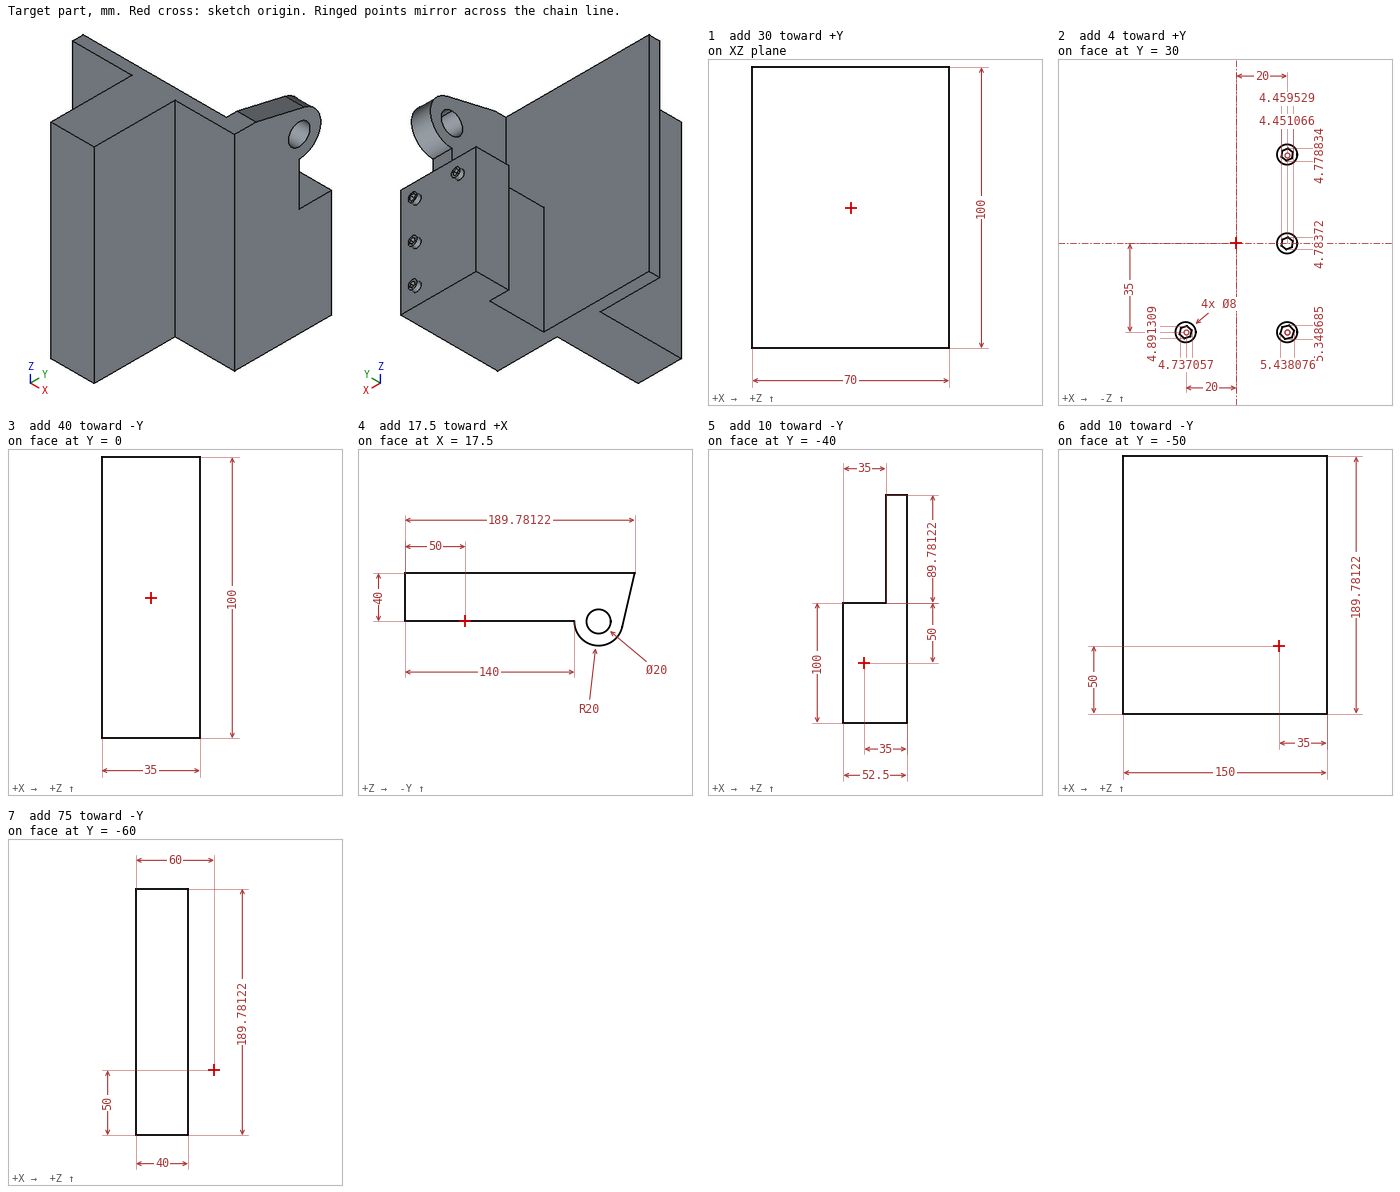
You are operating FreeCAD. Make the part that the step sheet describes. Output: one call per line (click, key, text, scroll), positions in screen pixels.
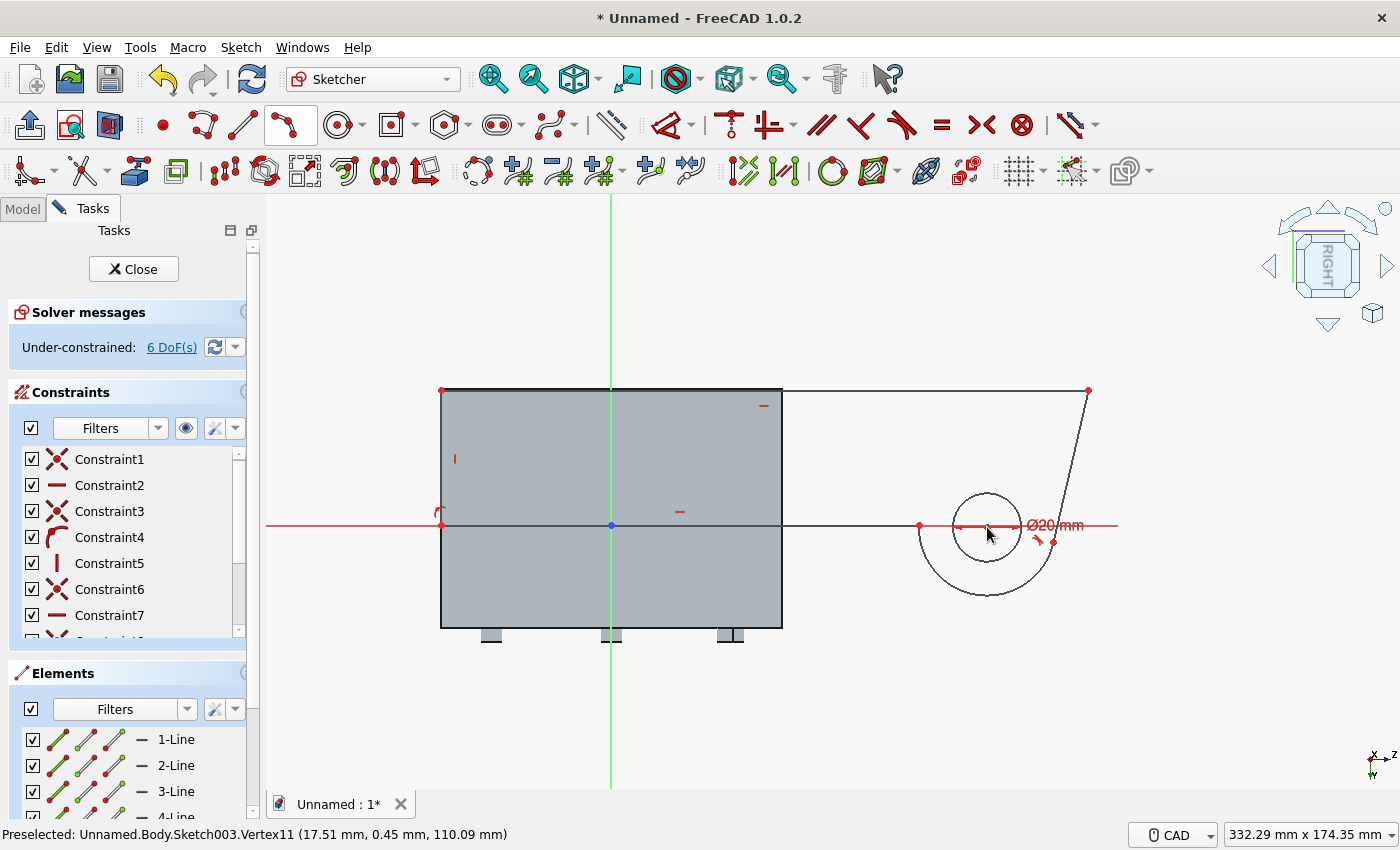
click(361, 526)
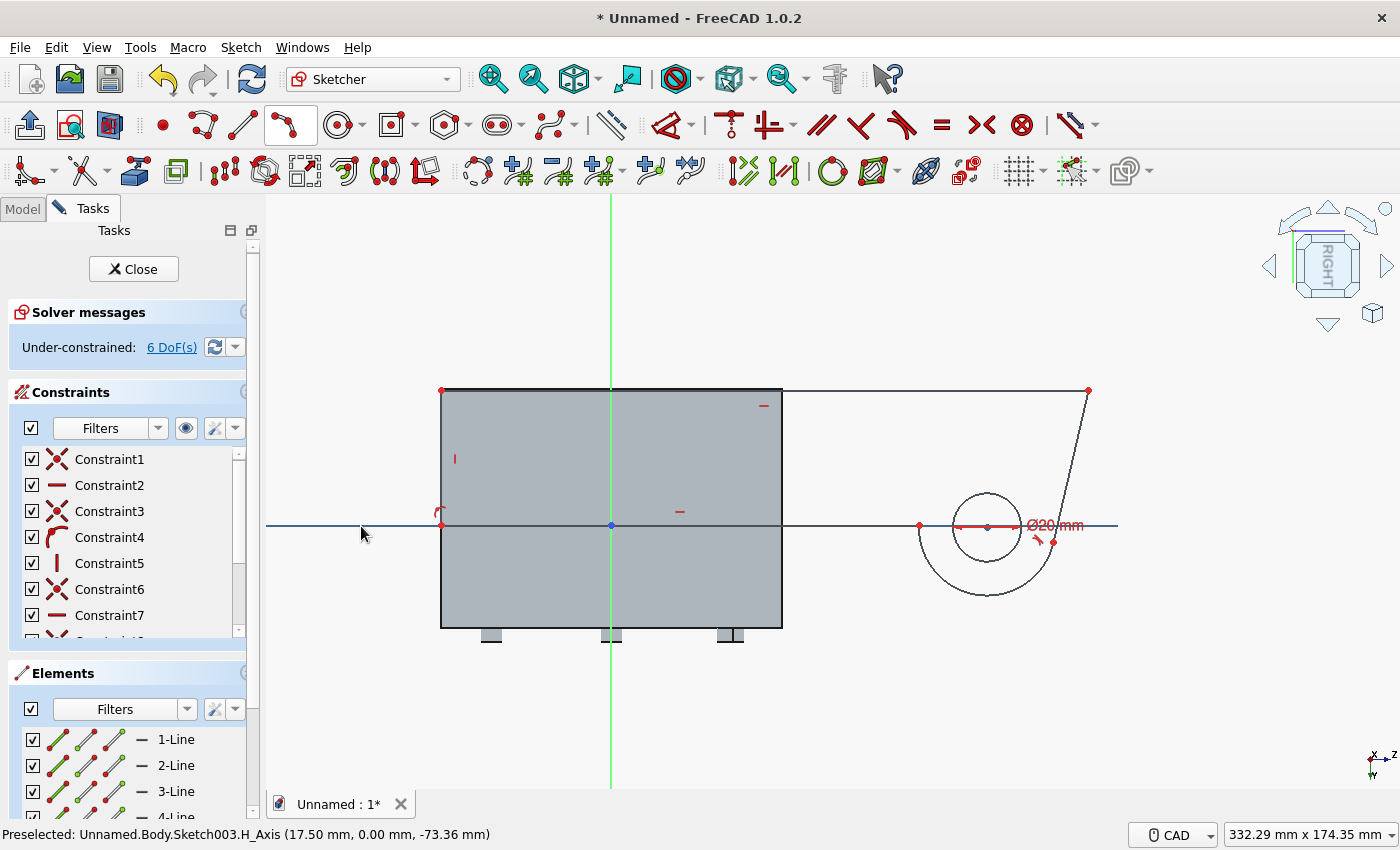
click(730, 126)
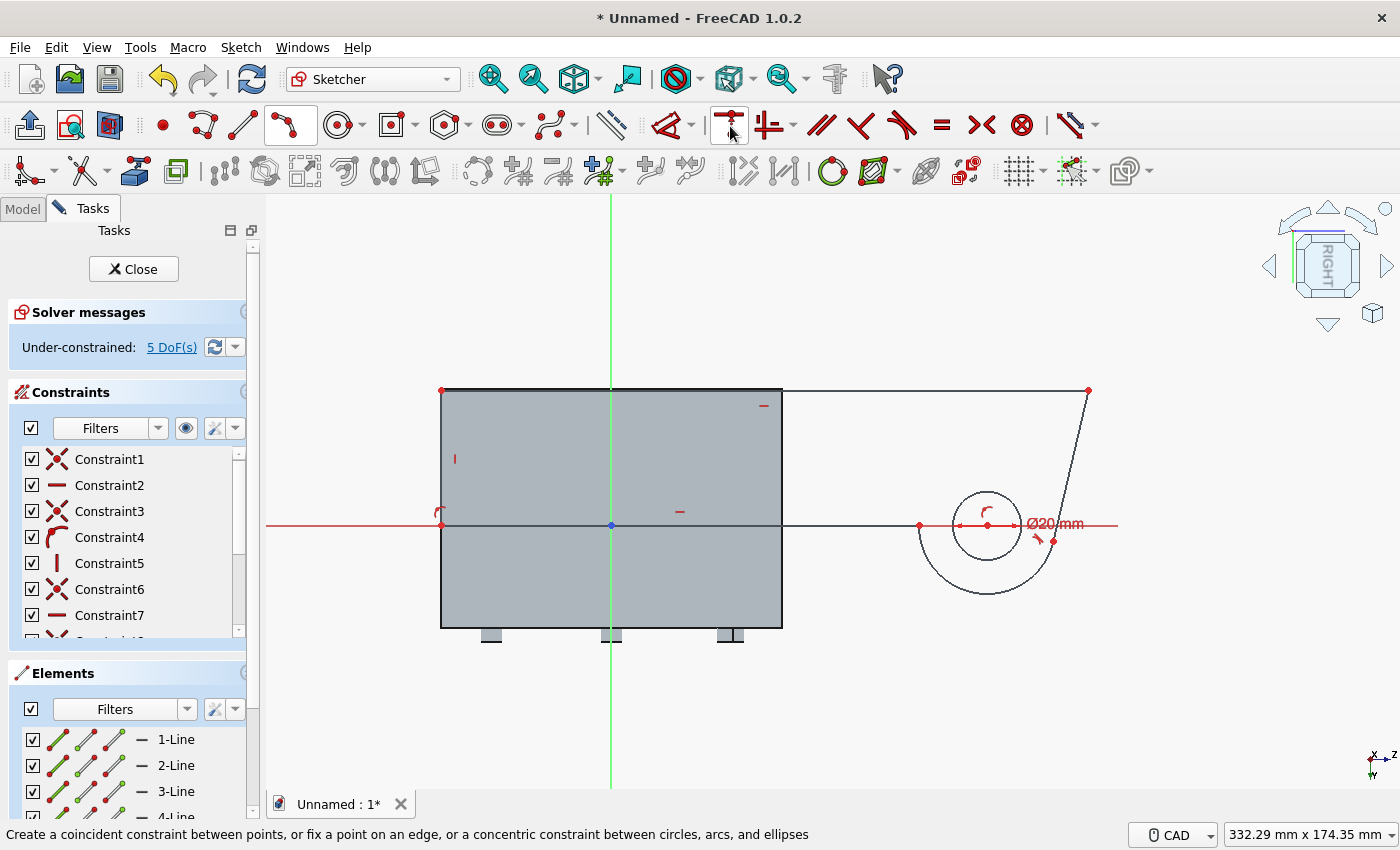
key(d)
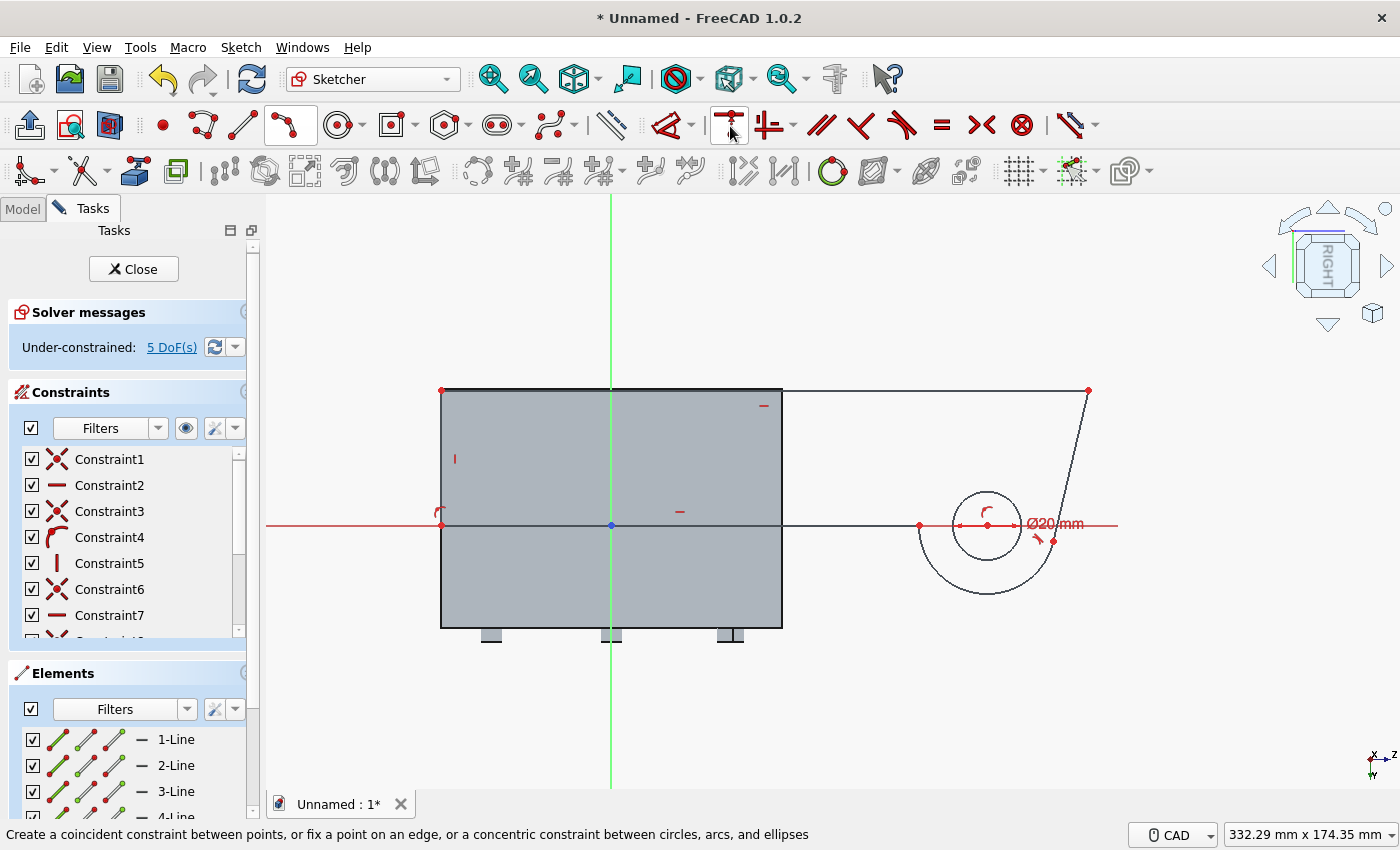
click(943, 578)
click(922, 602)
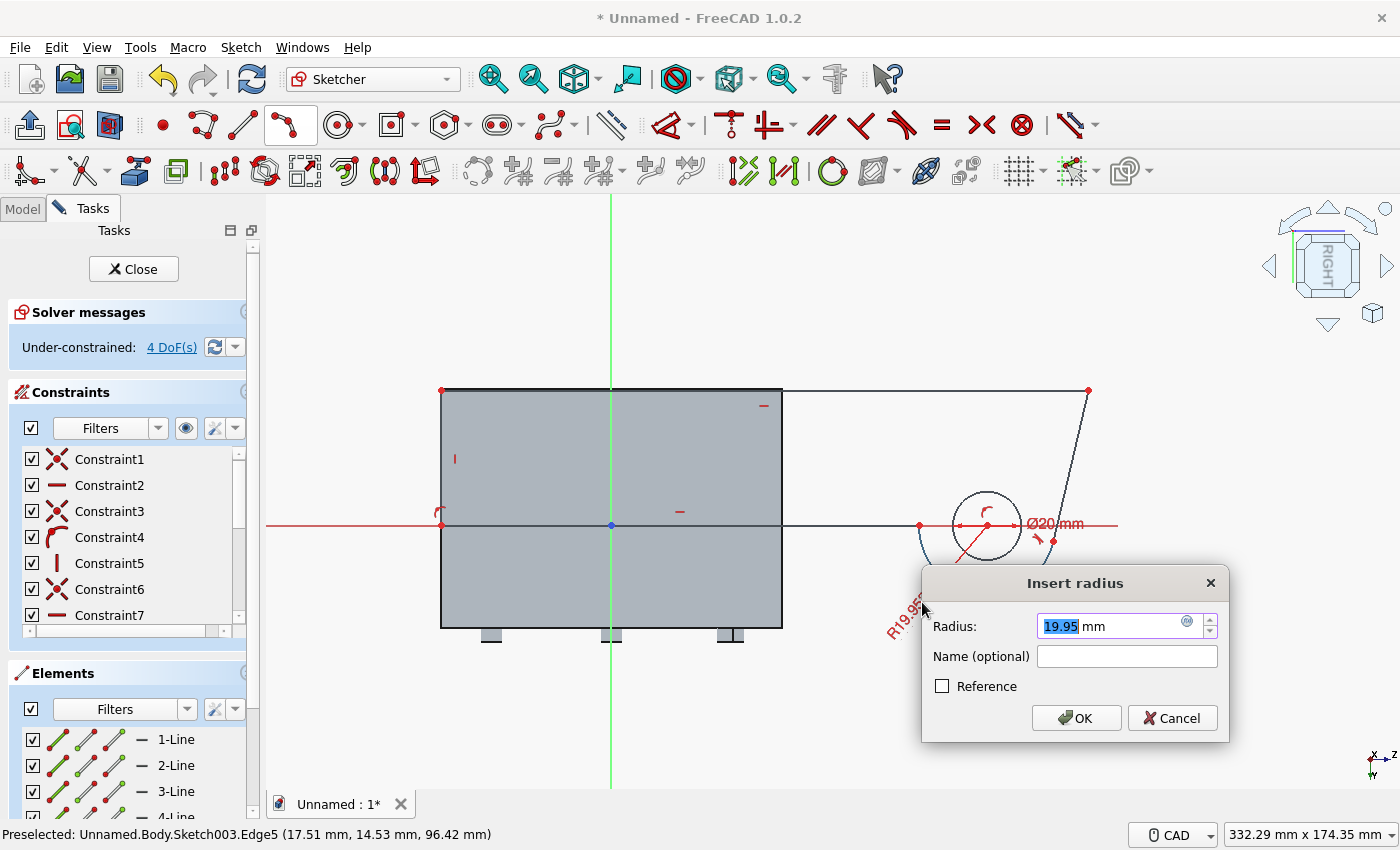
text(20)
key(Return)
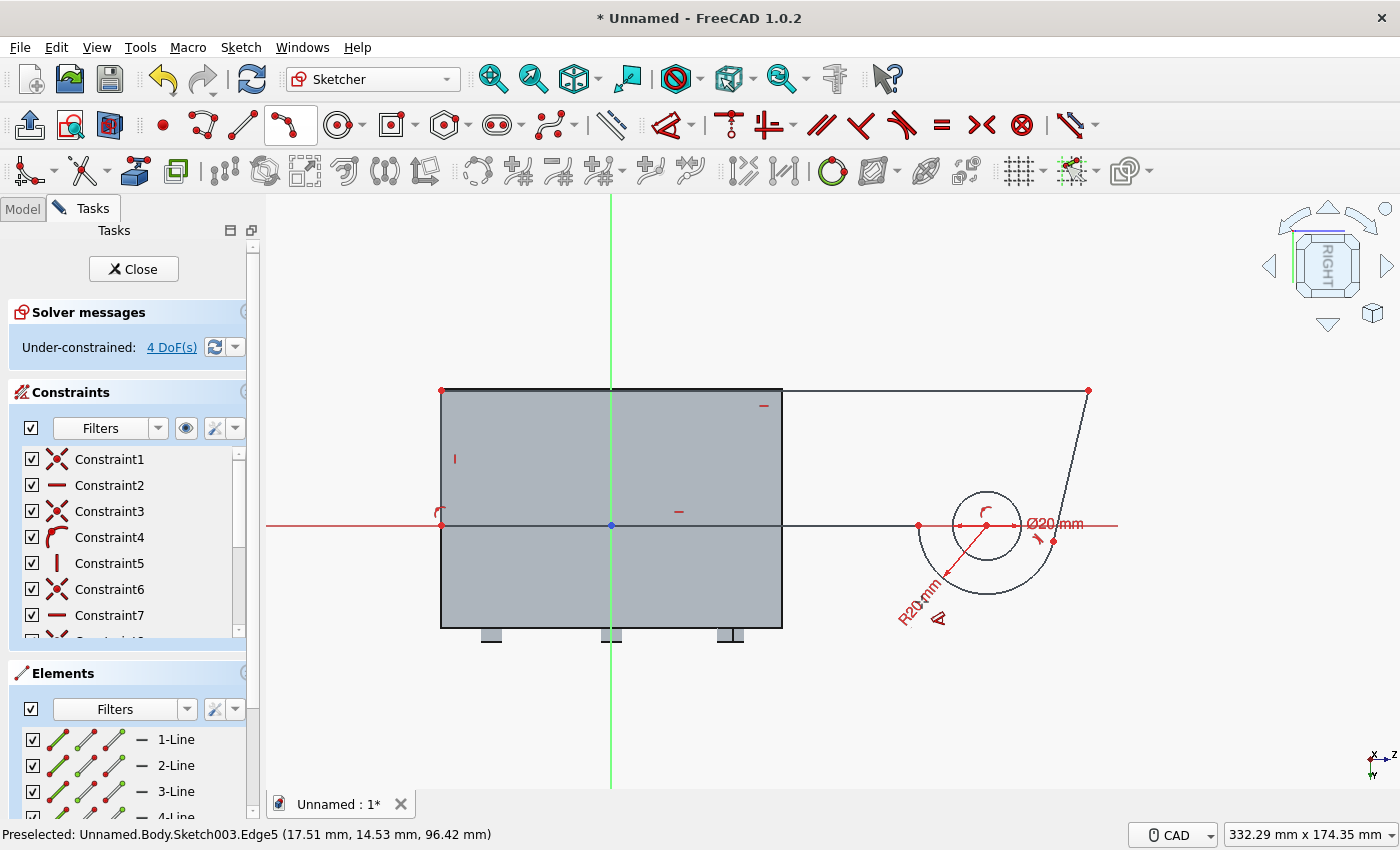
click(441, 431)
click(407, 458)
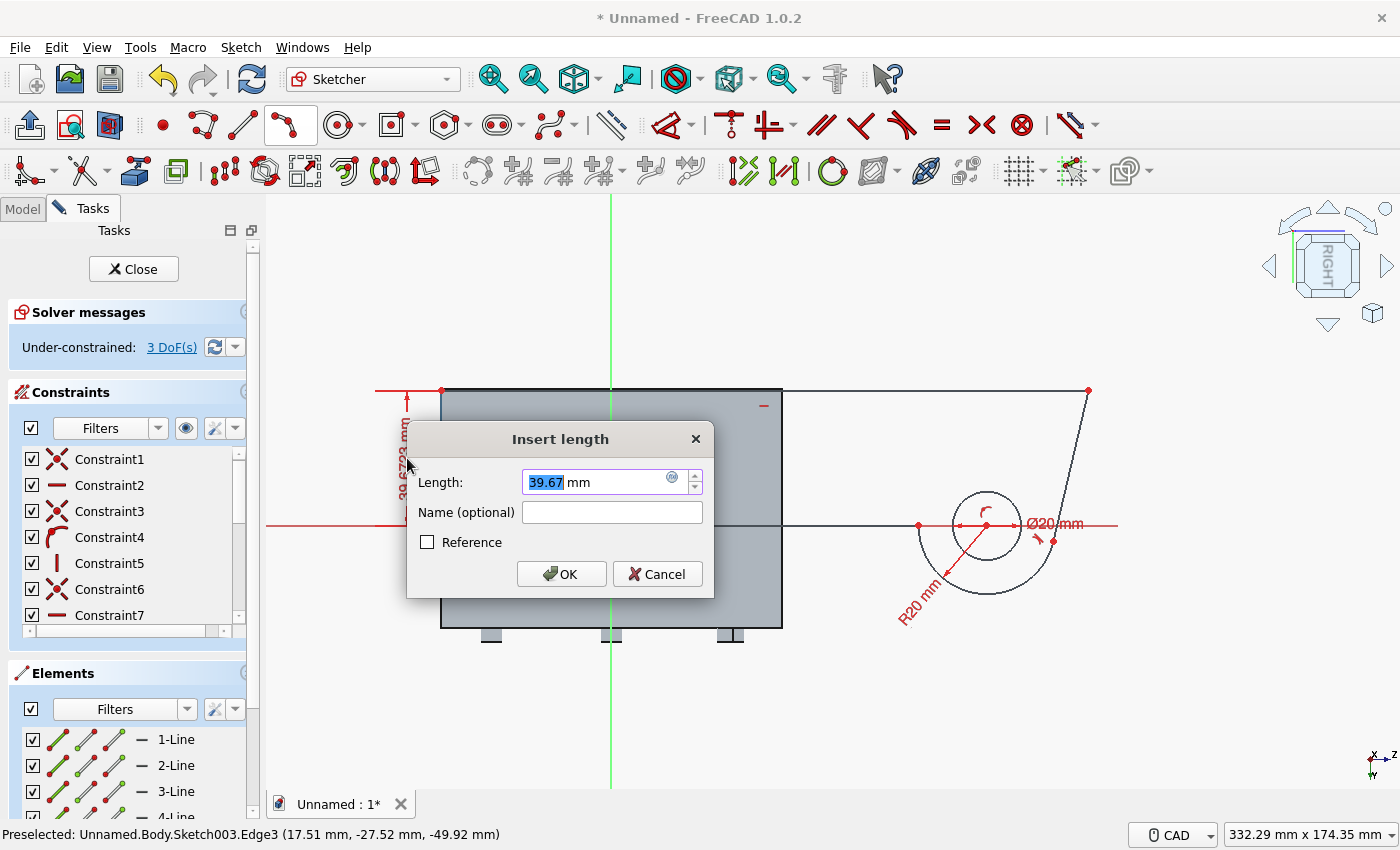
text(40)
key(Return)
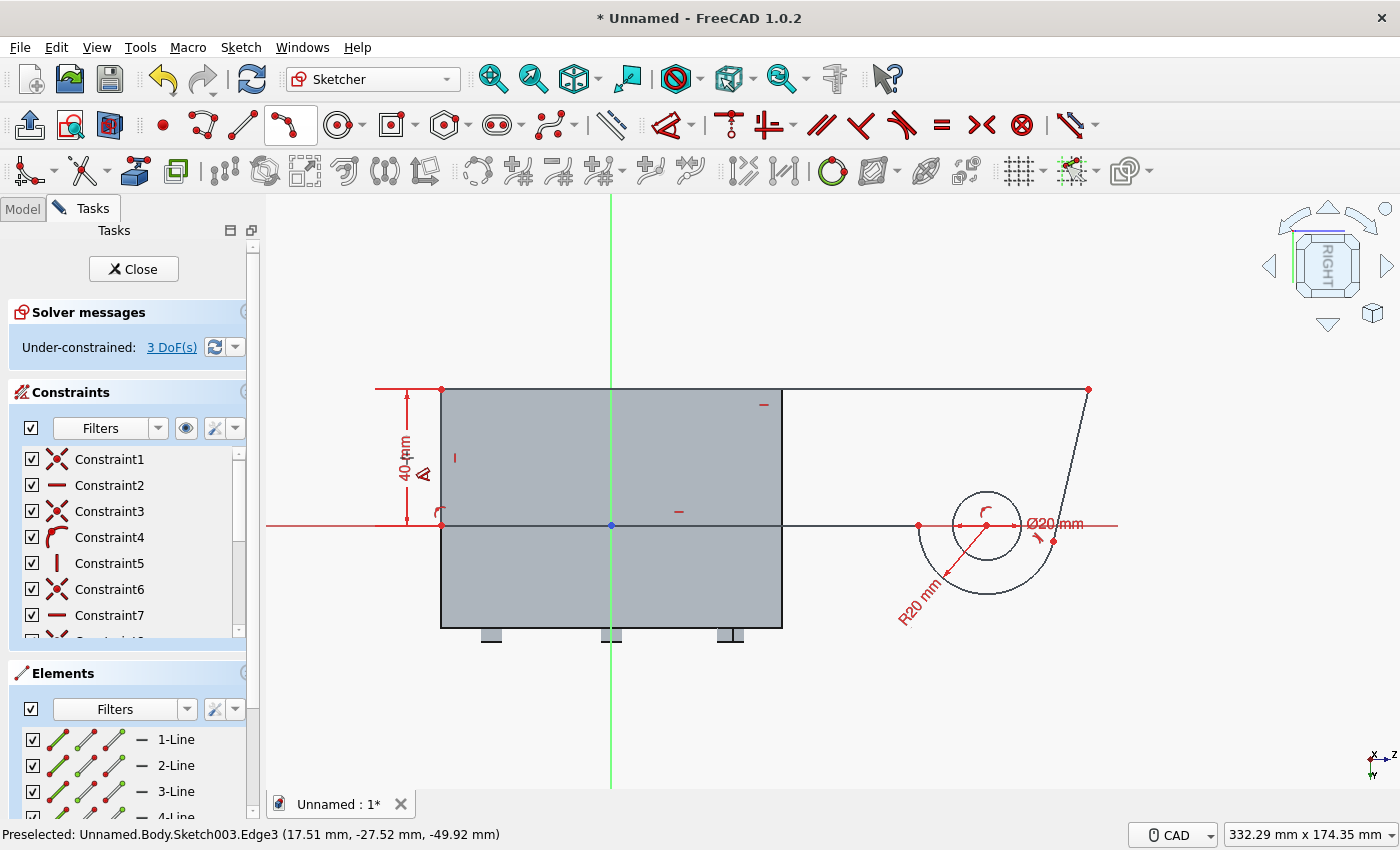
click(584, 526)
click(680, 560)